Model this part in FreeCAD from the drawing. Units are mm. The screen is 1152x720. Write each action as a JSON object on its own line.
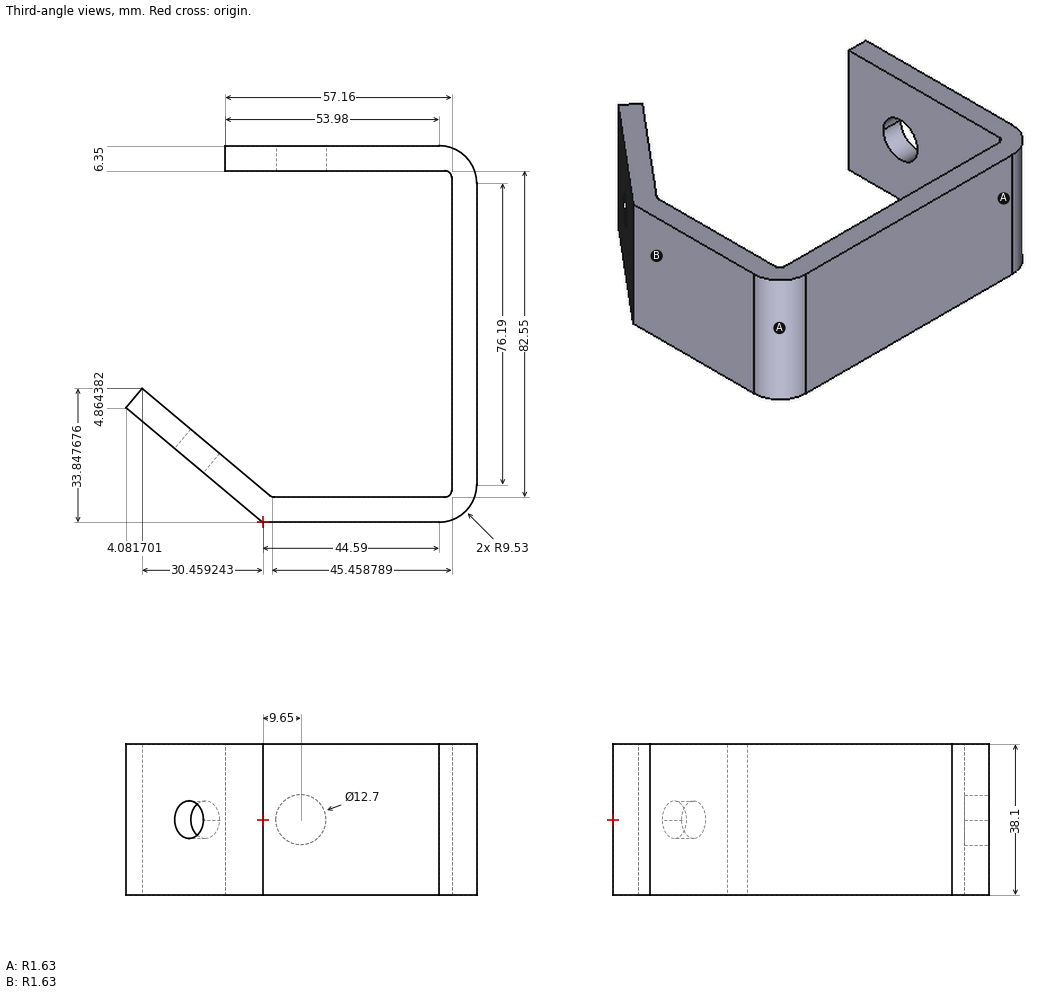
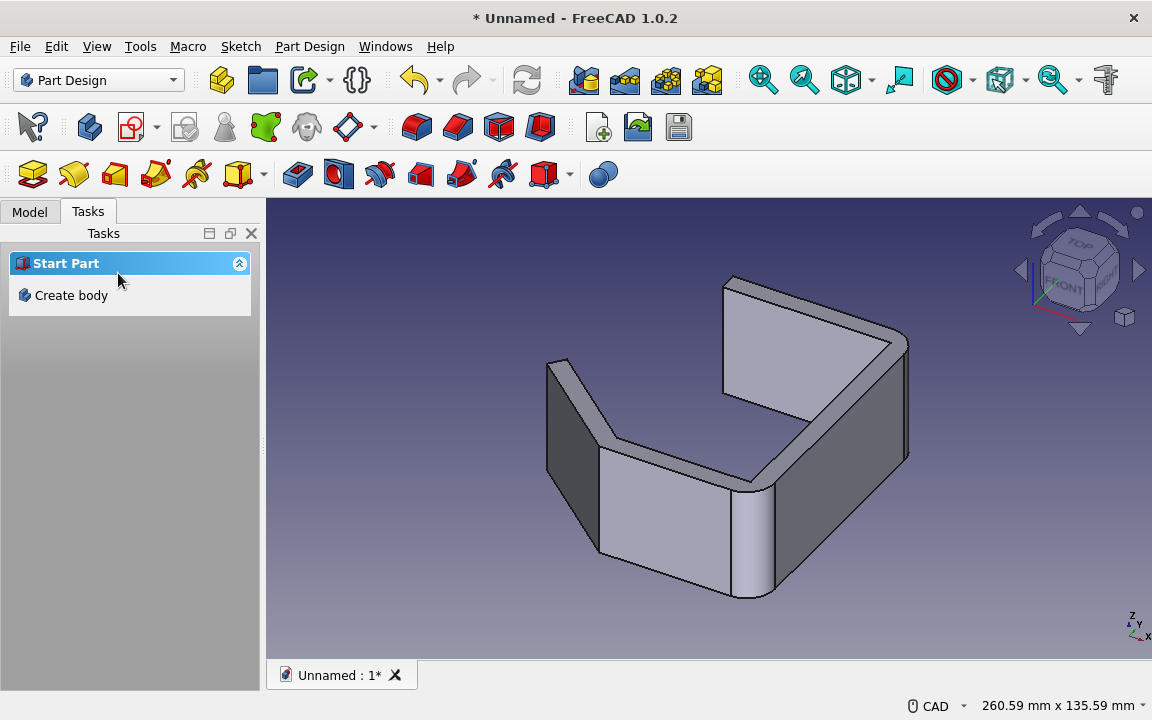
{"action": "key", "text": "4"}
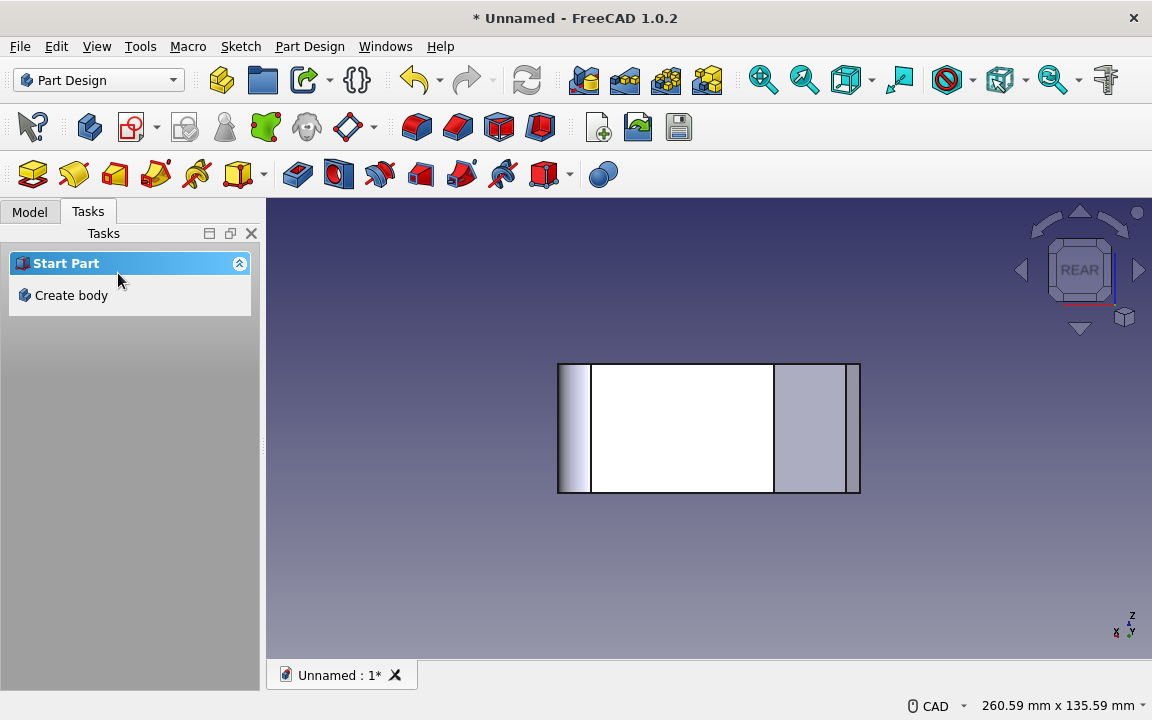
{"action": "left_click", "coordinate": [764, 80]}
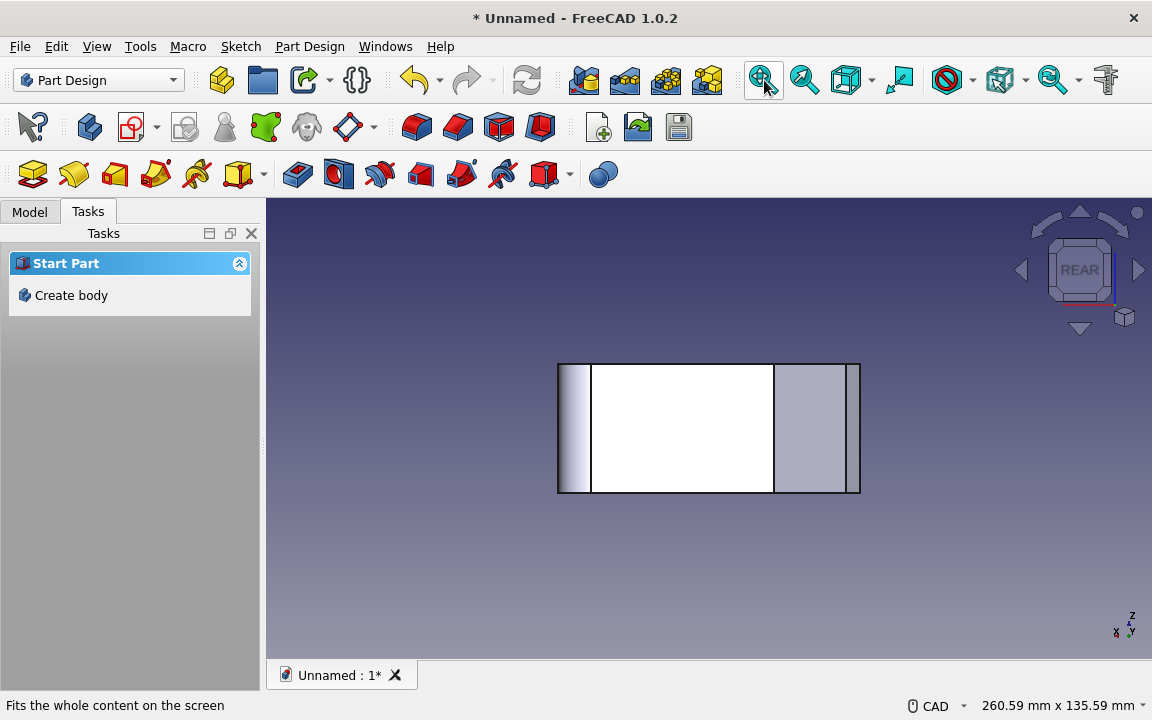
{"action": "left_click", "coordinate": [656, 428]}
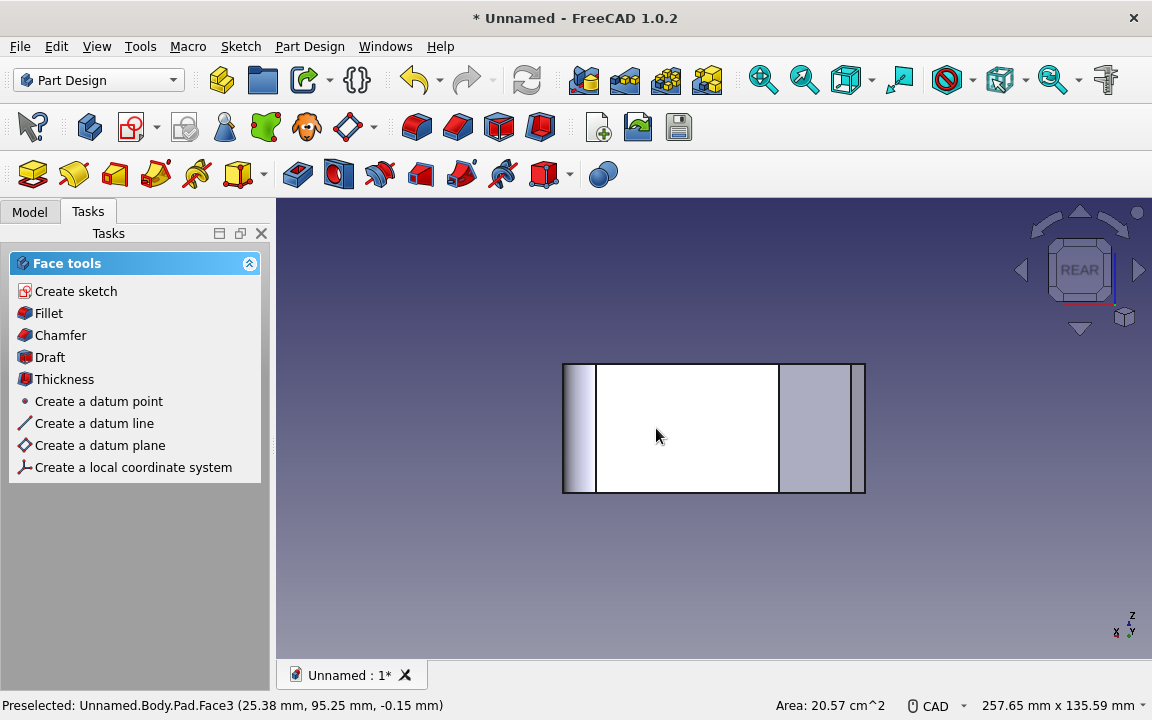
{"action": "left_click", "coordinate": [130, 128]}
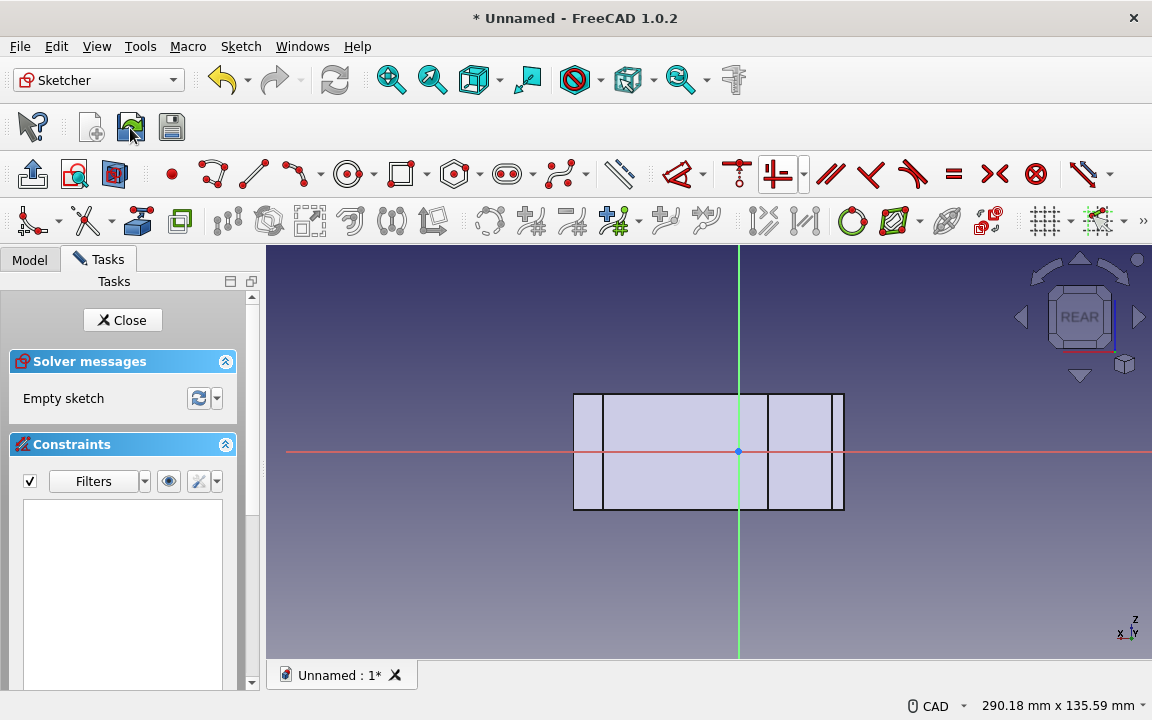
{"action": "scroll", "coordinate": [729, 452], "scroll_direction": "up", "scroll_amount": 9}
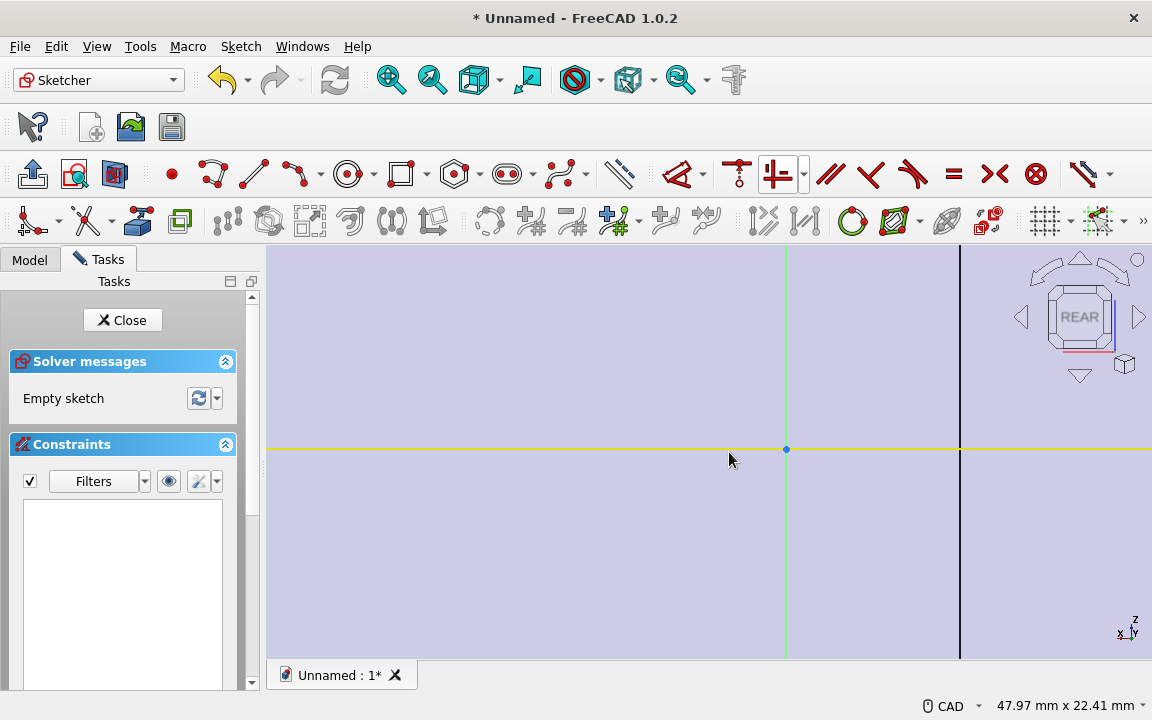
{"action": "key", "text": "g c"}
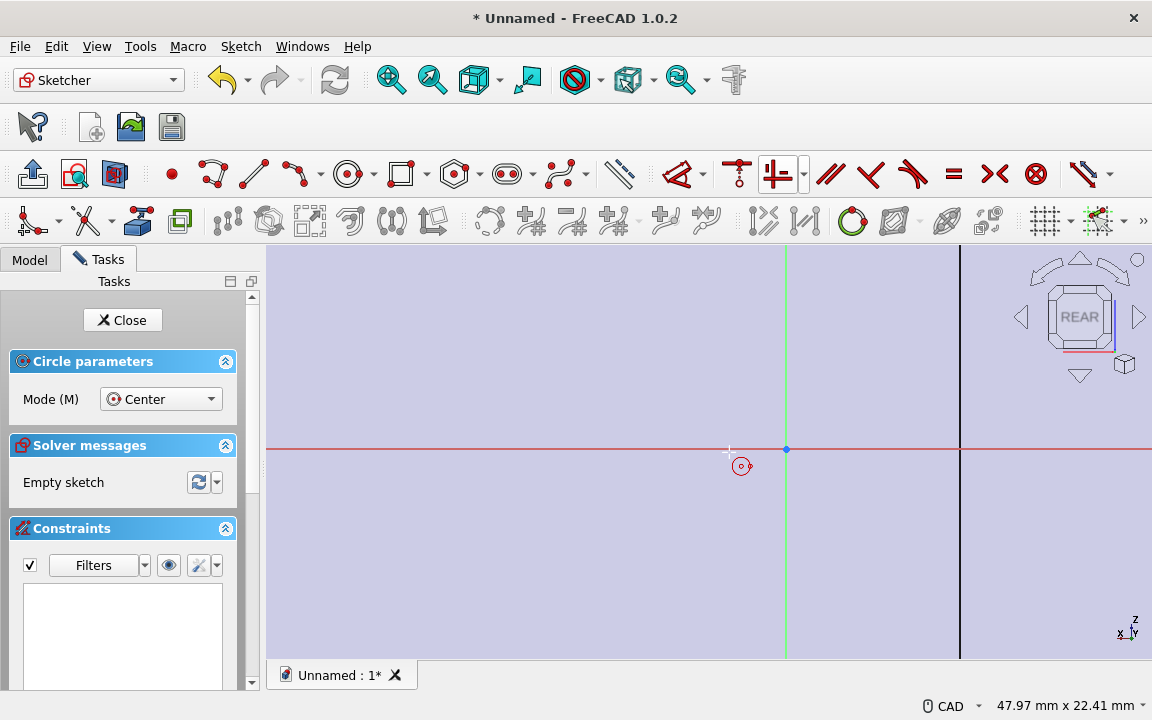
{"action": "left_click", "coordinate": [608, 449]}
{"action": "mouse_move", "coordinate": [691, 367]}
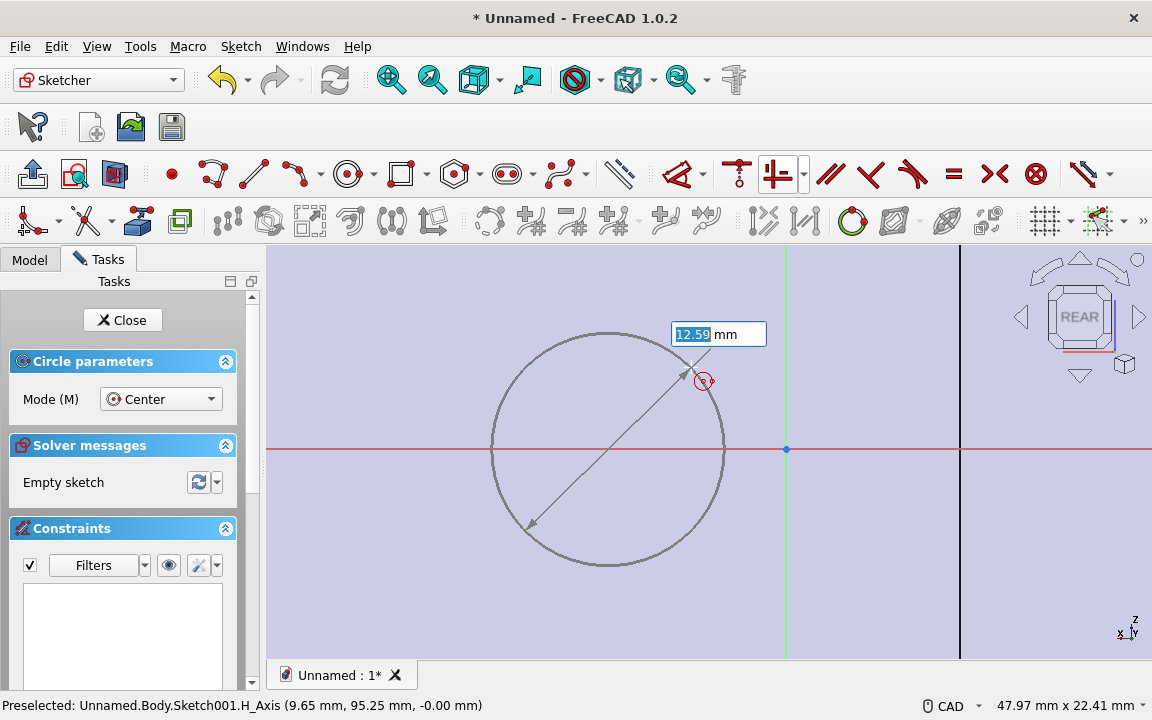
{"action": "type", "text": "12.7"}
{"action": "key", "text": "Return"}
{"action": "key", "text": "Escape"}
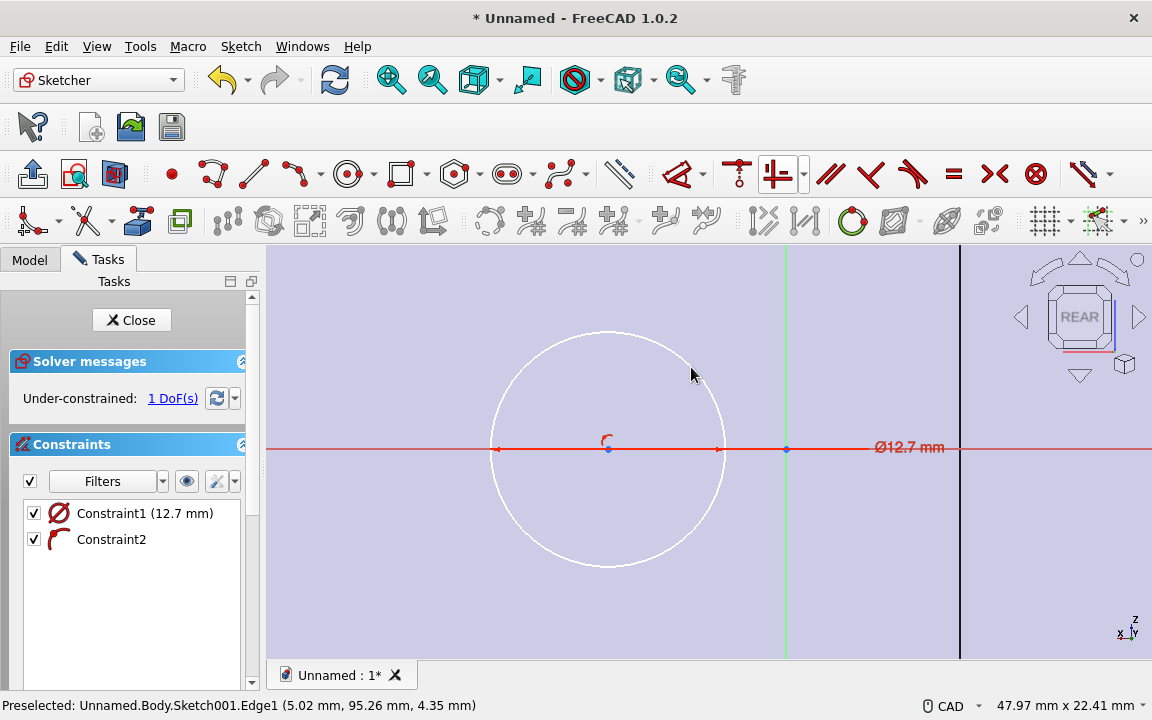
{"action": "key", "text": "d"}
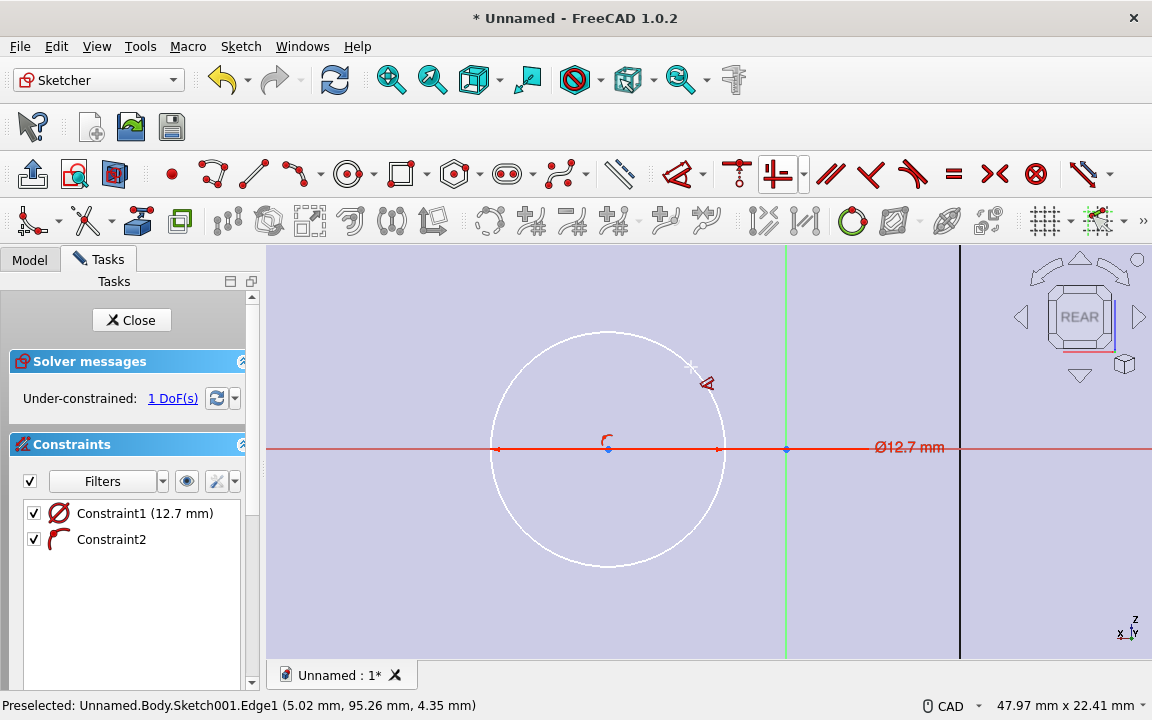
{"action": "left_click", "coordinate": [608, 449]}
{"action": "left_click", "coordinate": [697, 483]}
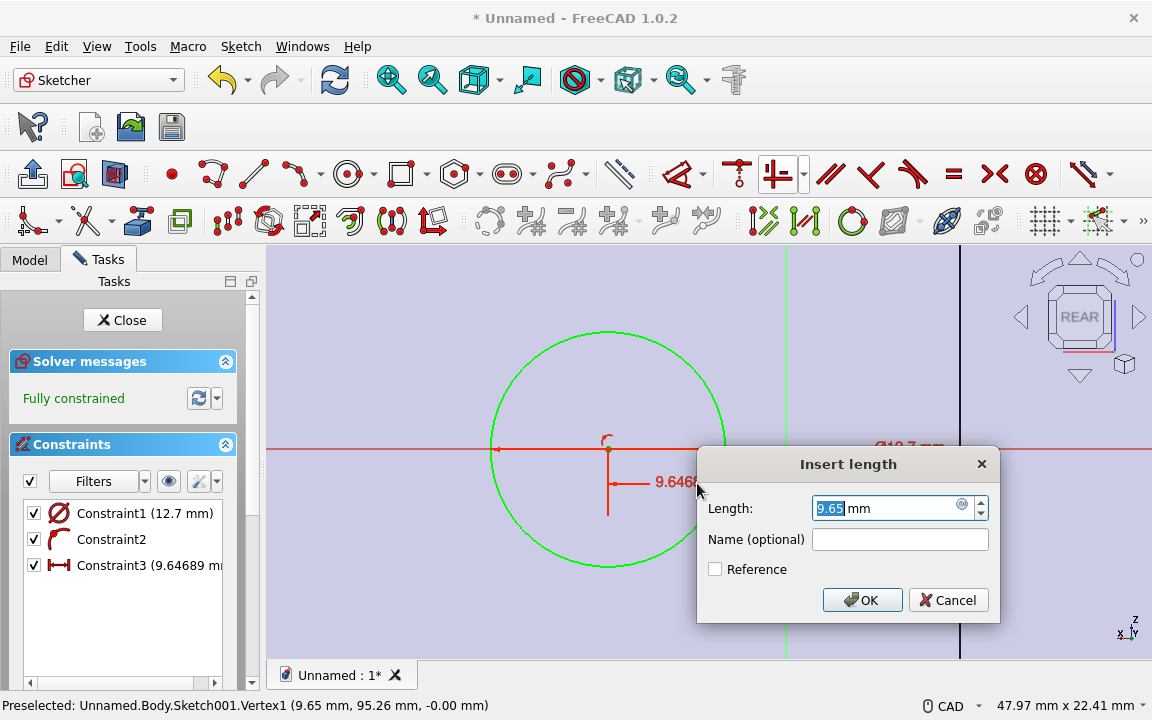
{"action": "type", "text": "9.65"}
{"action": "key", "text": "Return"}
{"action": "key", "text": "Escape"}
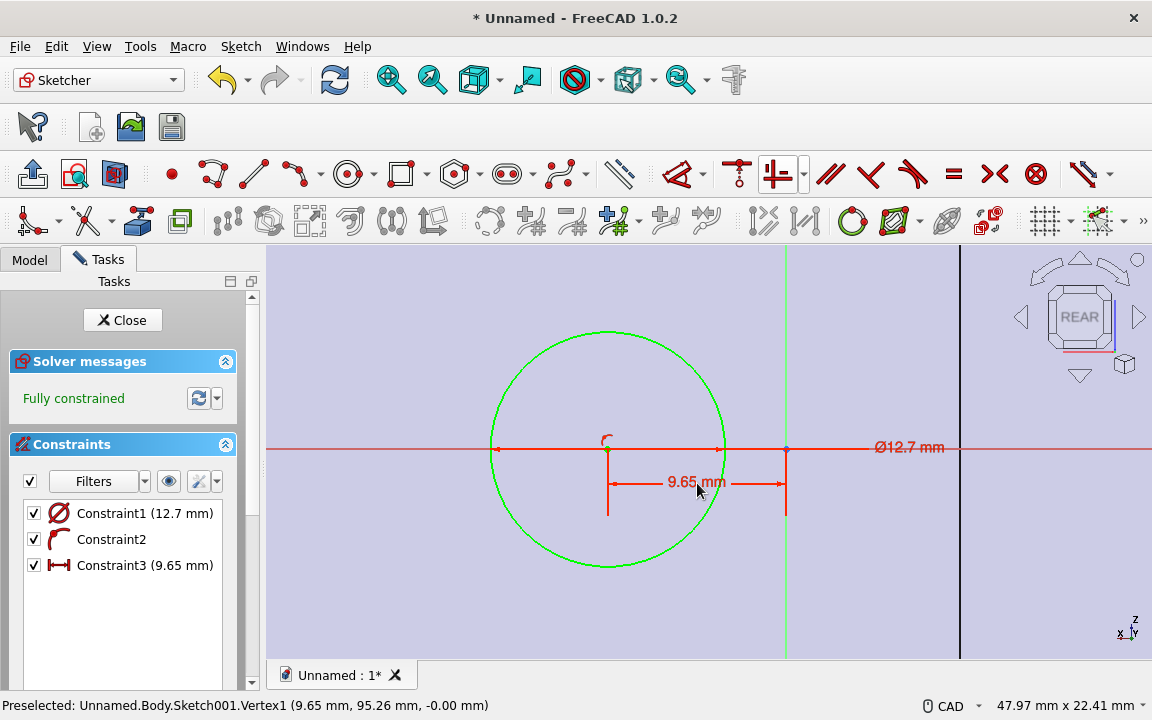
{"action": "left_click", "coordinate": [123, 320]}